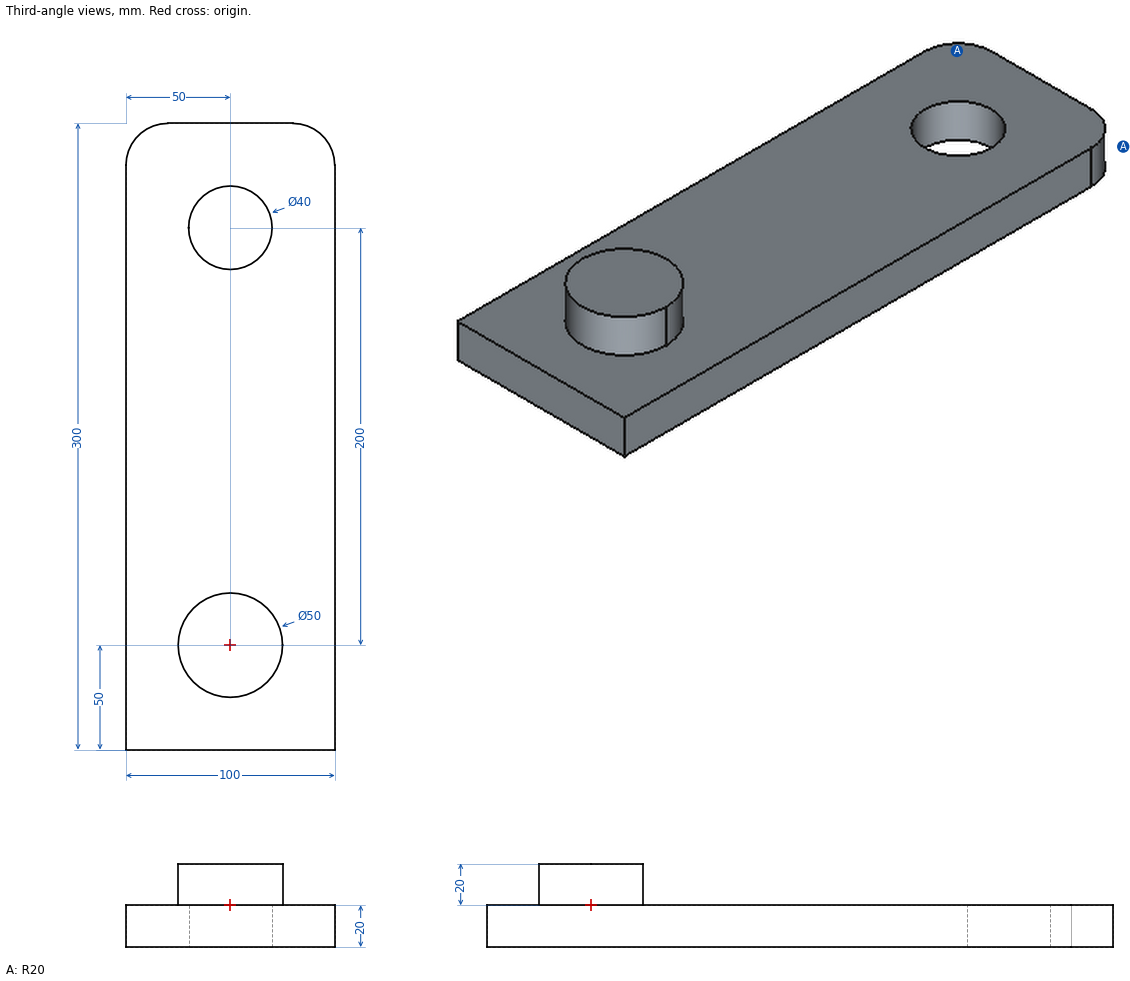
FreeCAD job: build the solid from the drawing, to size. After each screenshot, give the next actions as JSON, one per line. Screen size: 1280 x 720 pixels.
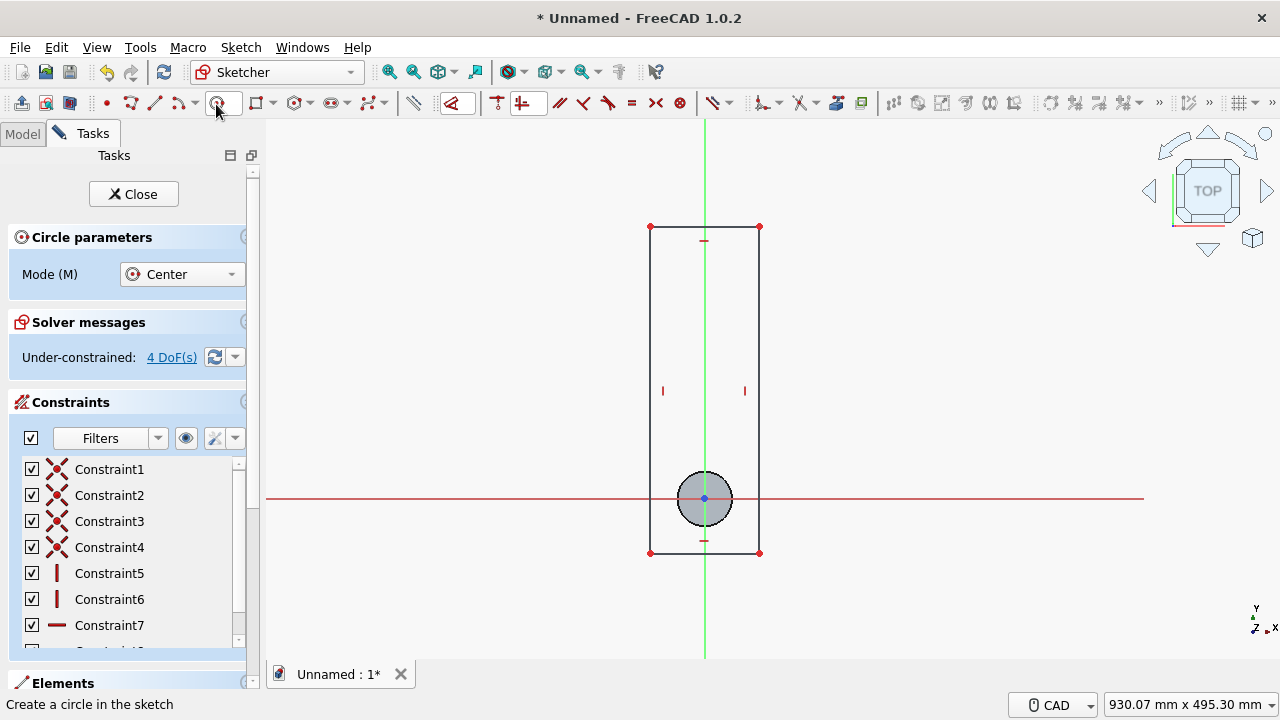
{"action": "left_click", "coordinate": [705, 281]}
{"action": "left_click", "coordinate": [720, 265]}
{"action": "key", "text": "Escape"}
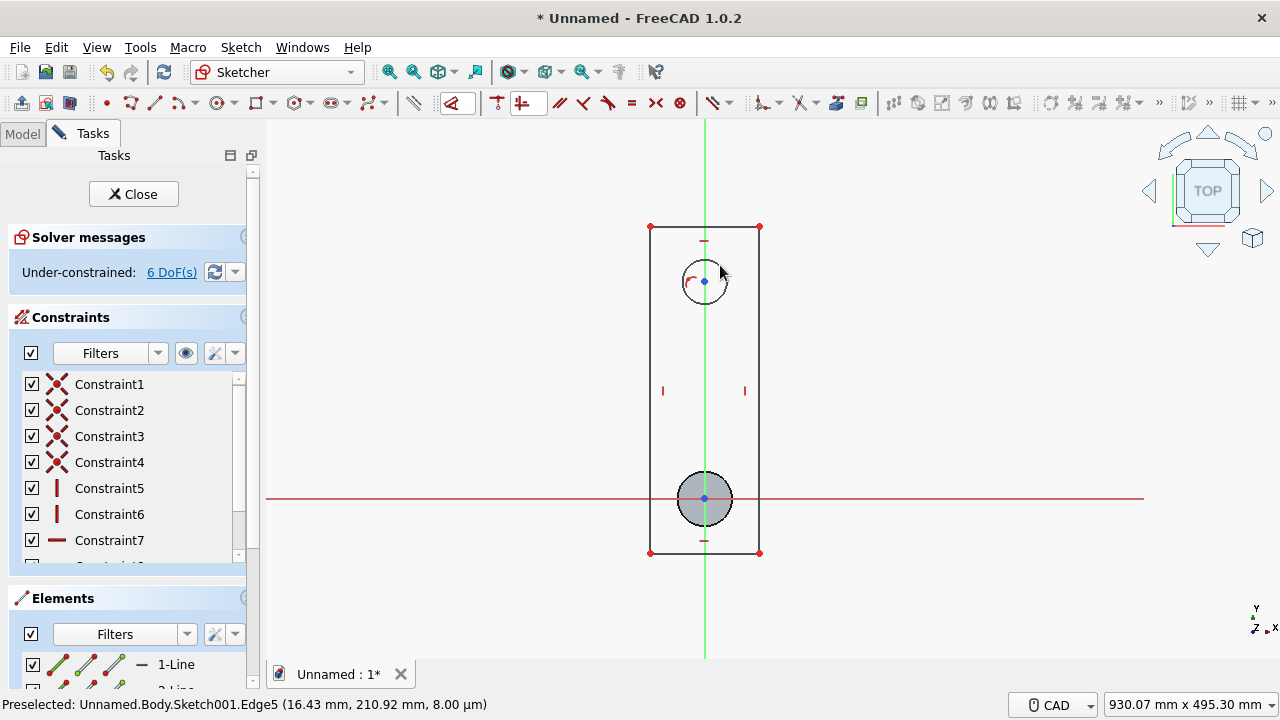
{"action": "left_click", "coordinate": [720, 266]}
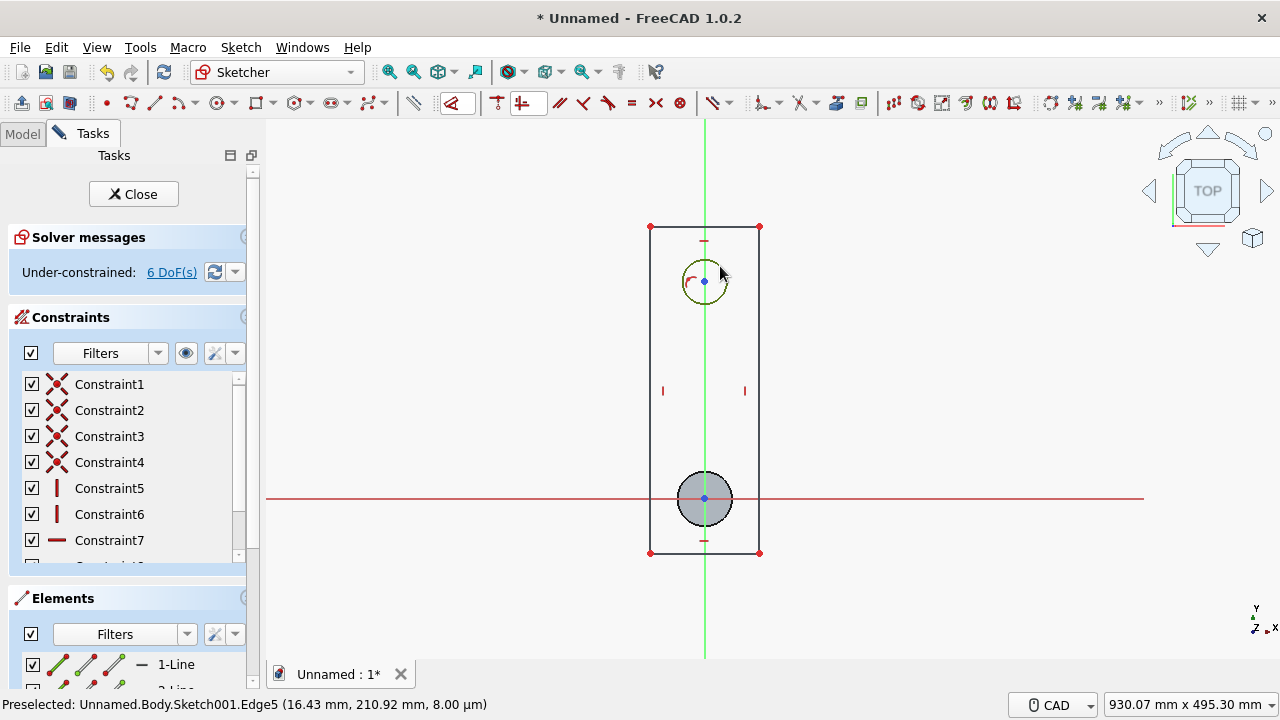
{"action": "left_click", "coordinate": [470, 104]}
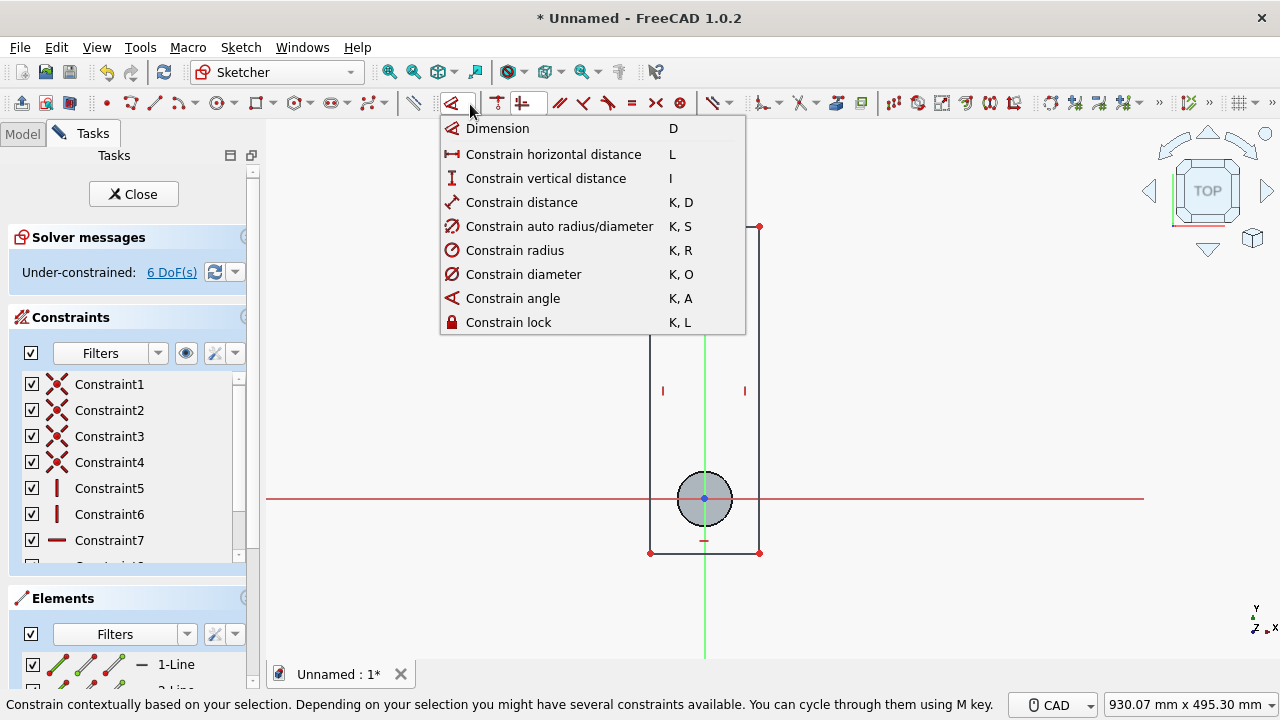
{"action": "left_click", "coordinate": [593, 274]}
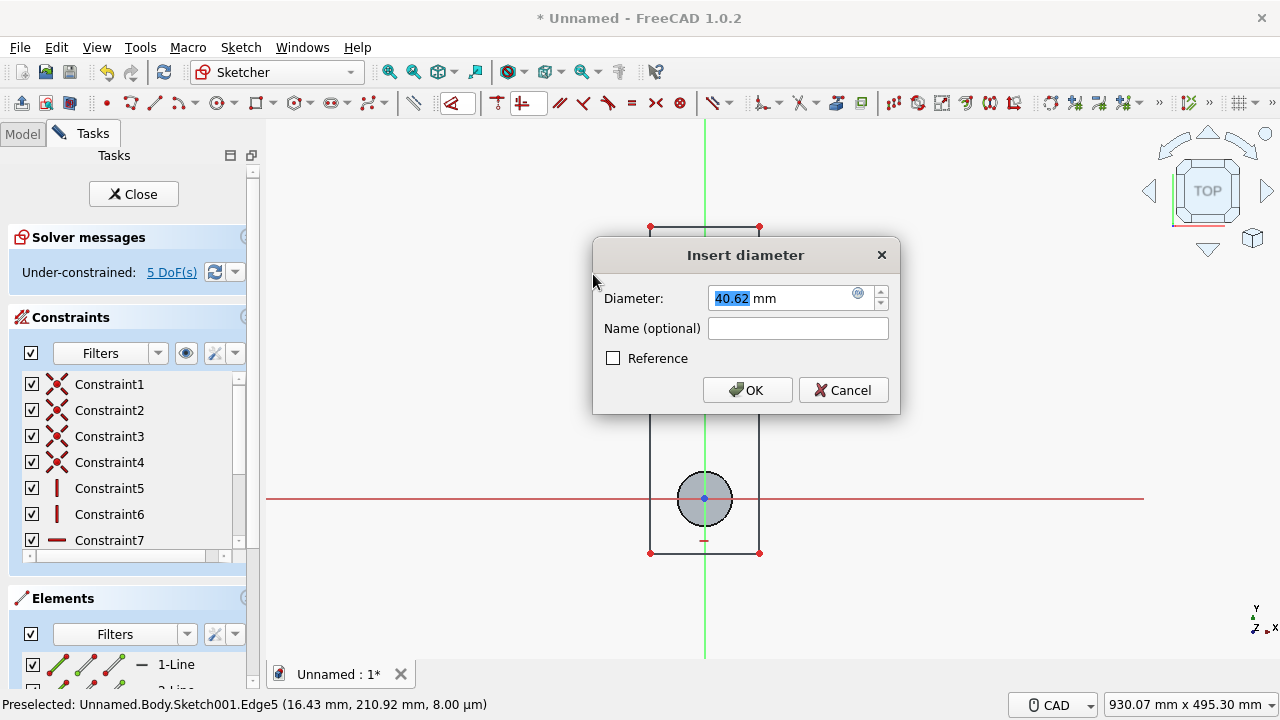
{"action": "type", "text": "40"}
{"action": "key", "text": "Return"}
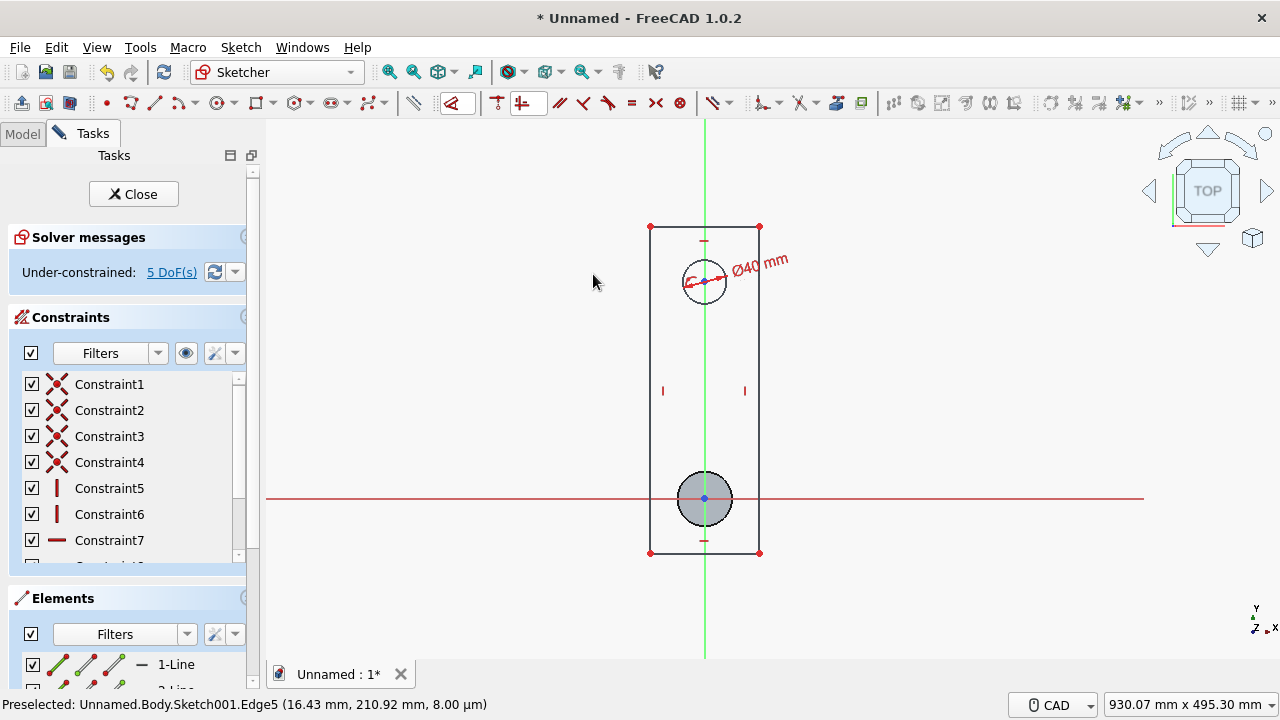
{"action": "left_click", "coordinate": [650, 325]}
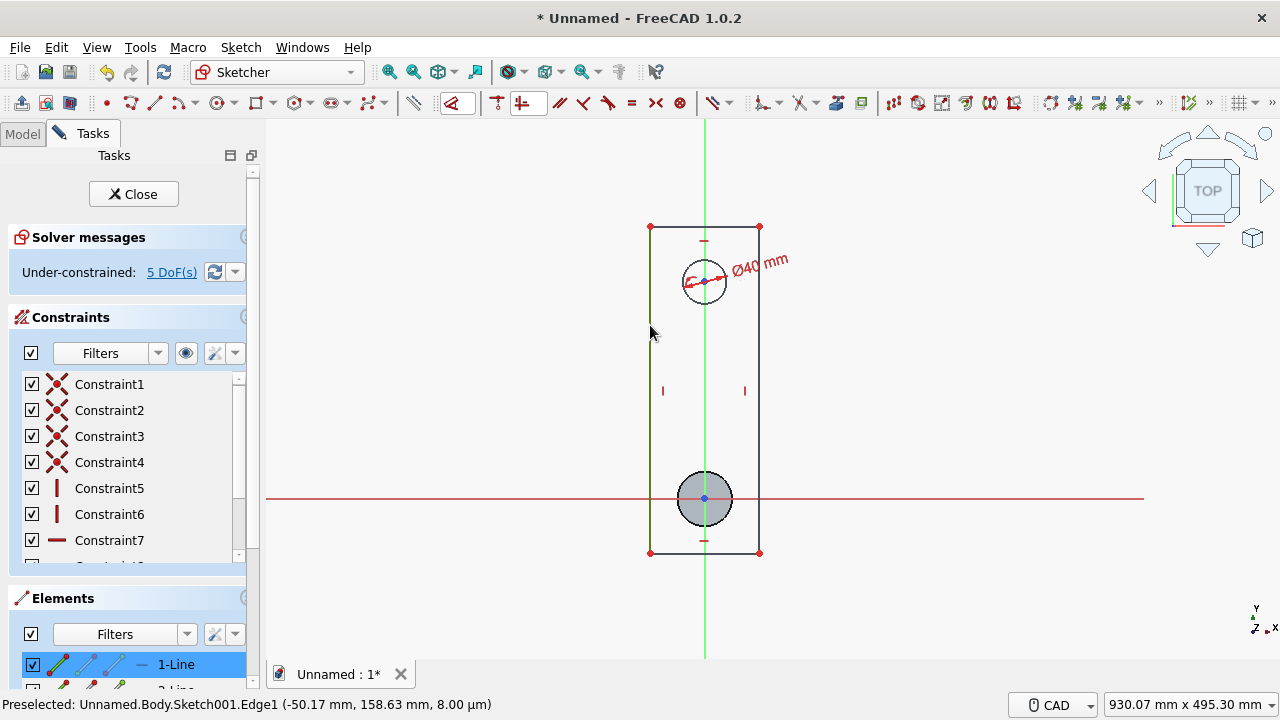
{"action": "left_click", "coordinate": [470, 104]}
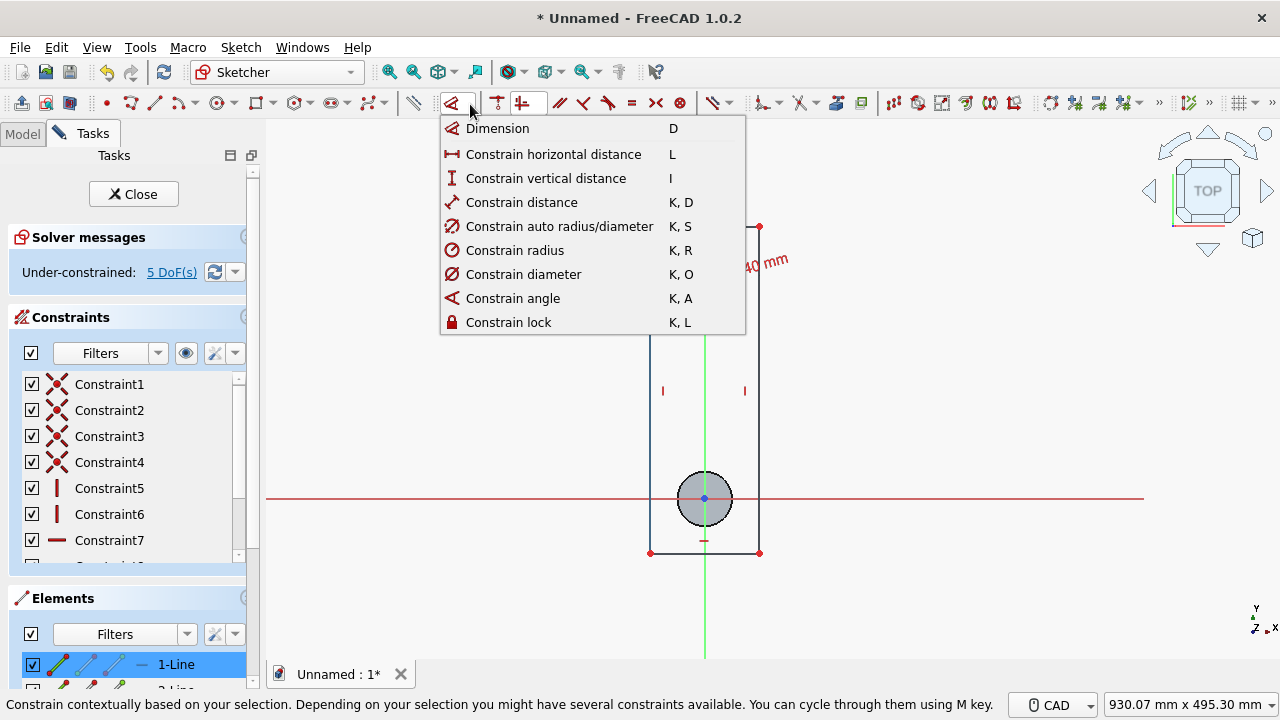
{"action": "left_click", "coordinate": [593, 178]}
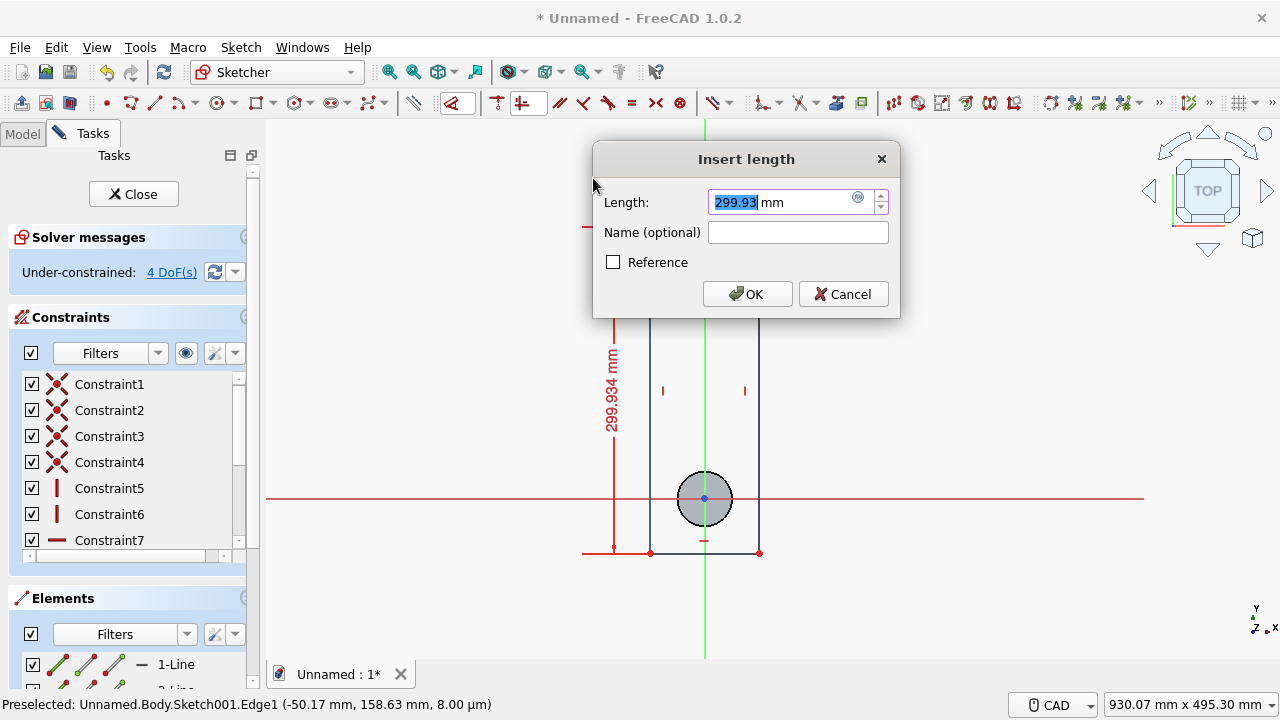
{"action": "type", "text": "300"}
{"action": "key", "text": "Return"}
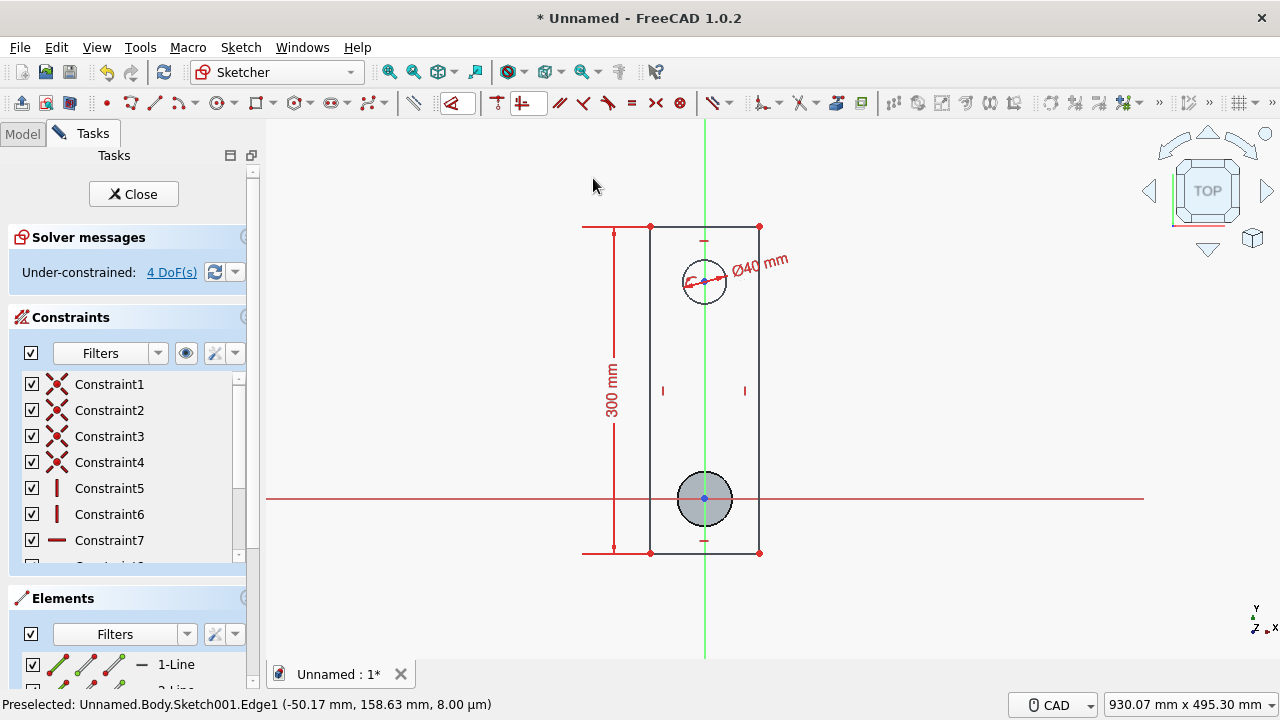
{"action": "left_click", "coordinate": [683, 554]}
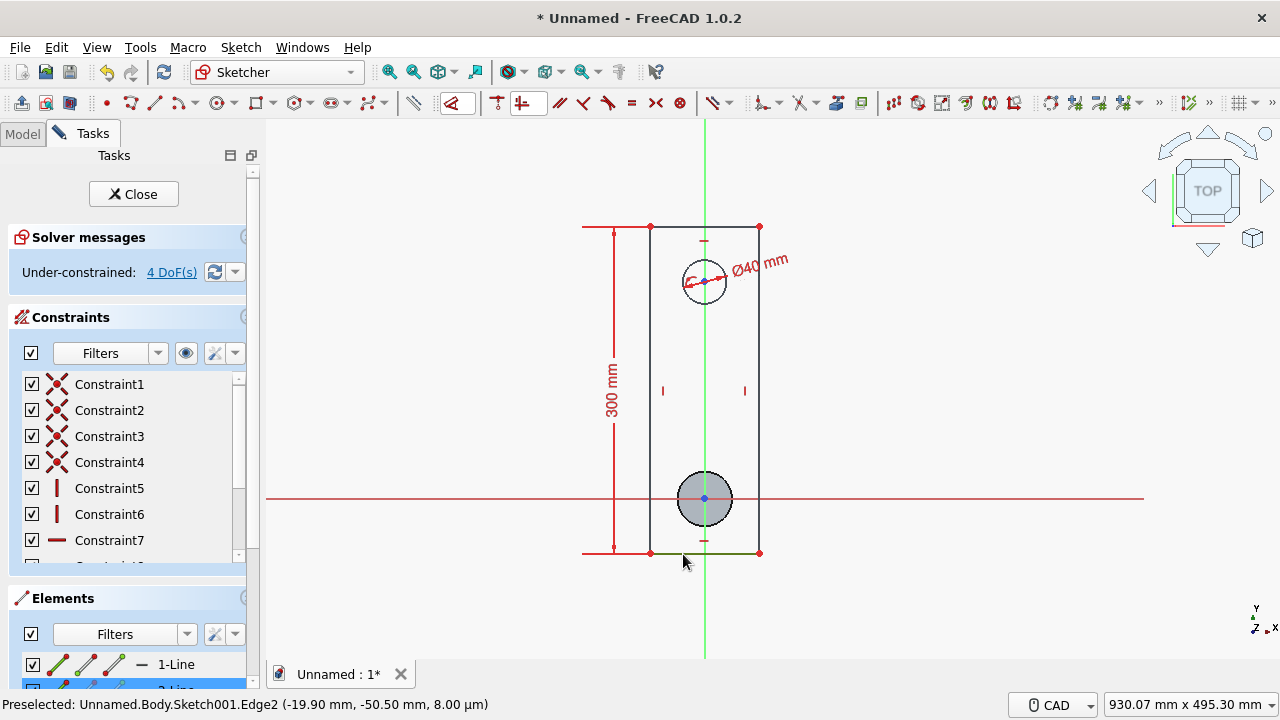
{"action": "key", "text": "l"}